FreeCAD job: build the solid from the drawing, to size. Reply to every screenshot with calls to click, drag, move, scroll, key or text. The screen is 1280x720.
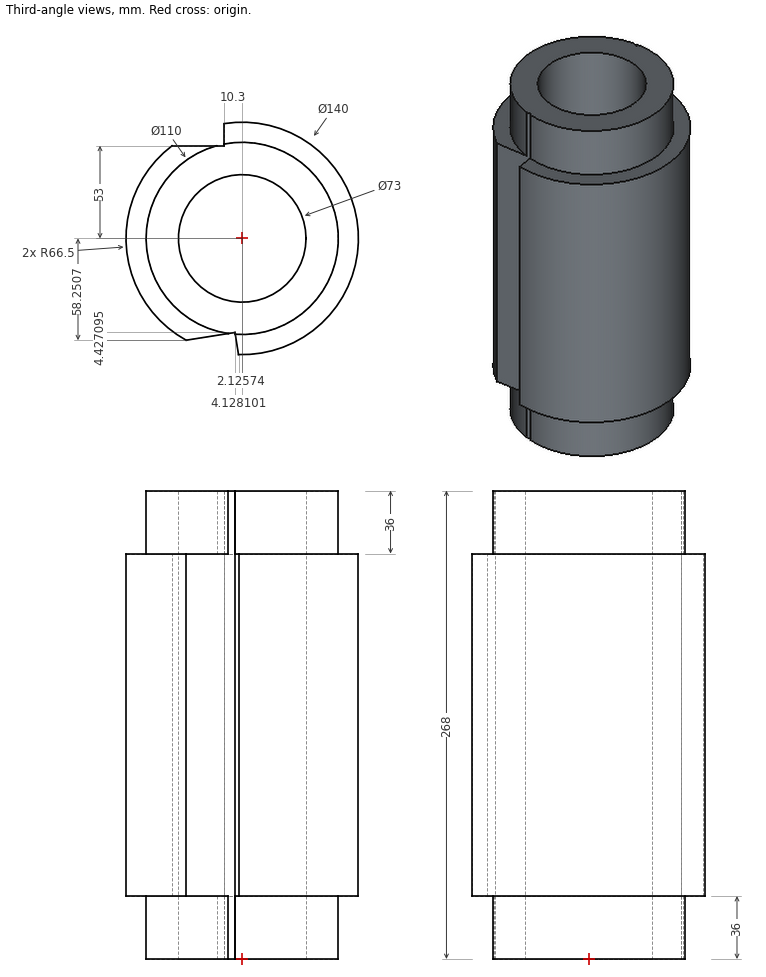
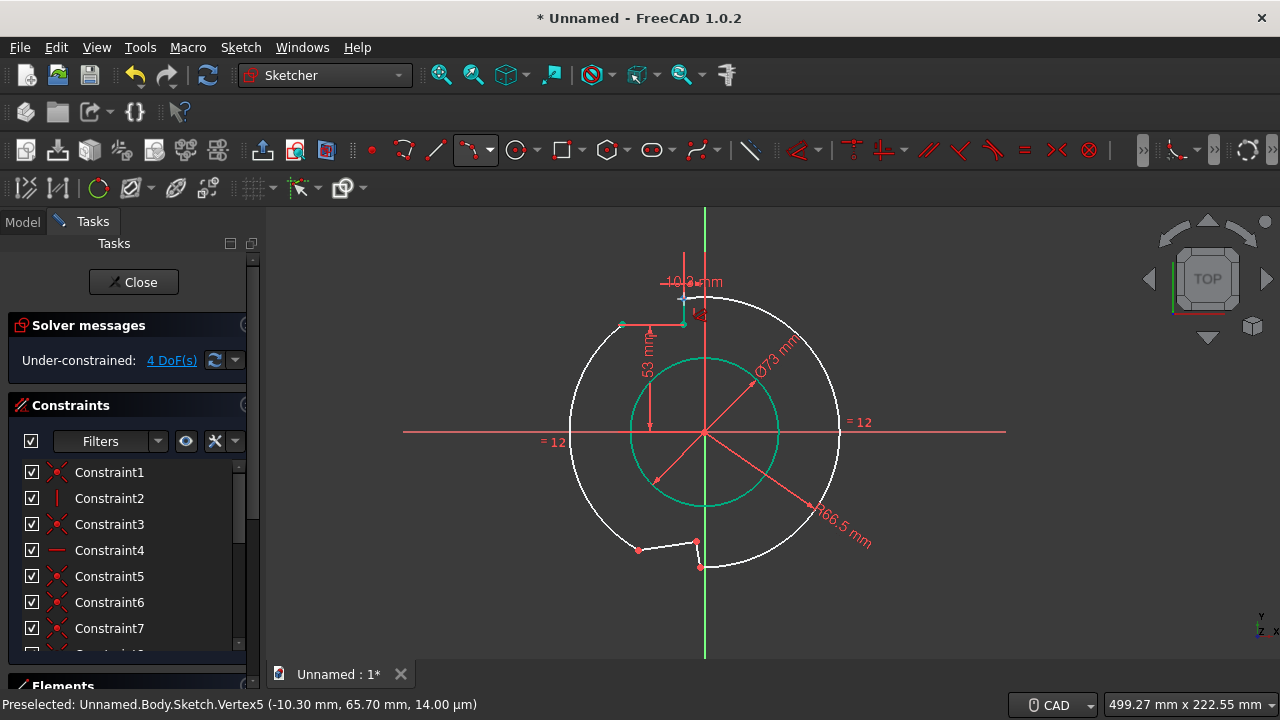
click(639, 550)
click(605, 491)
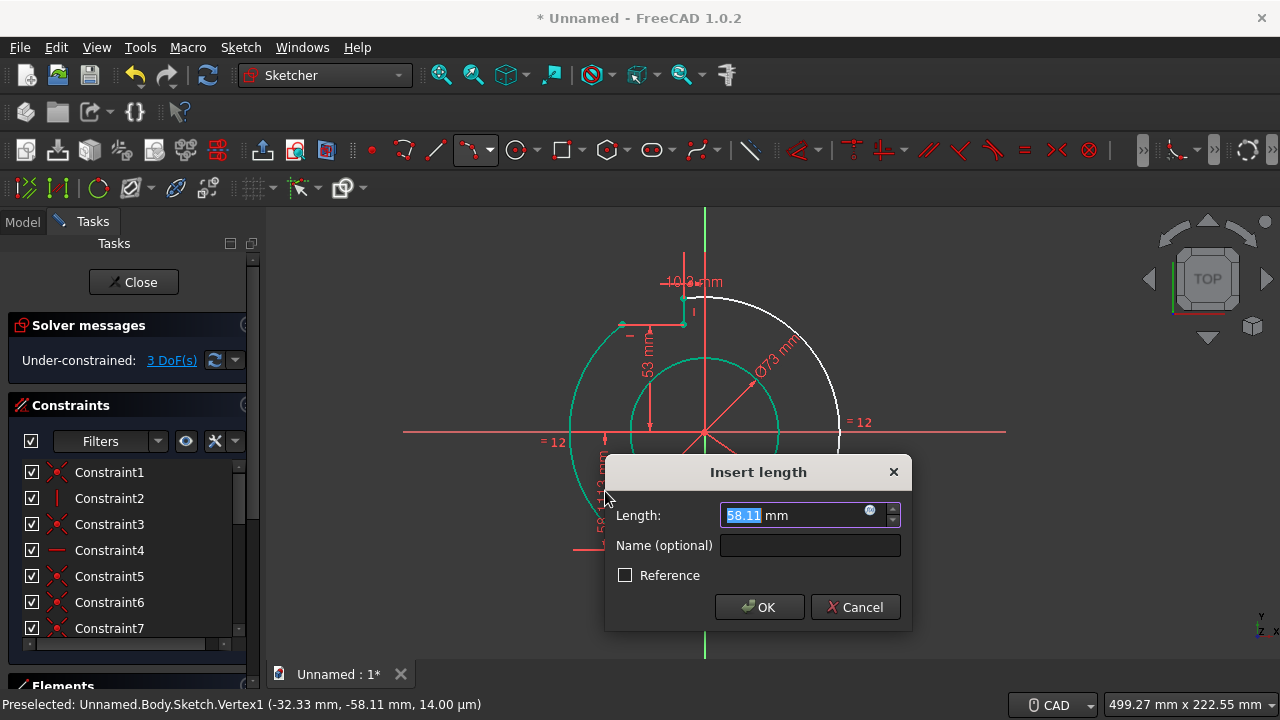
text(58.2507)
key(Return)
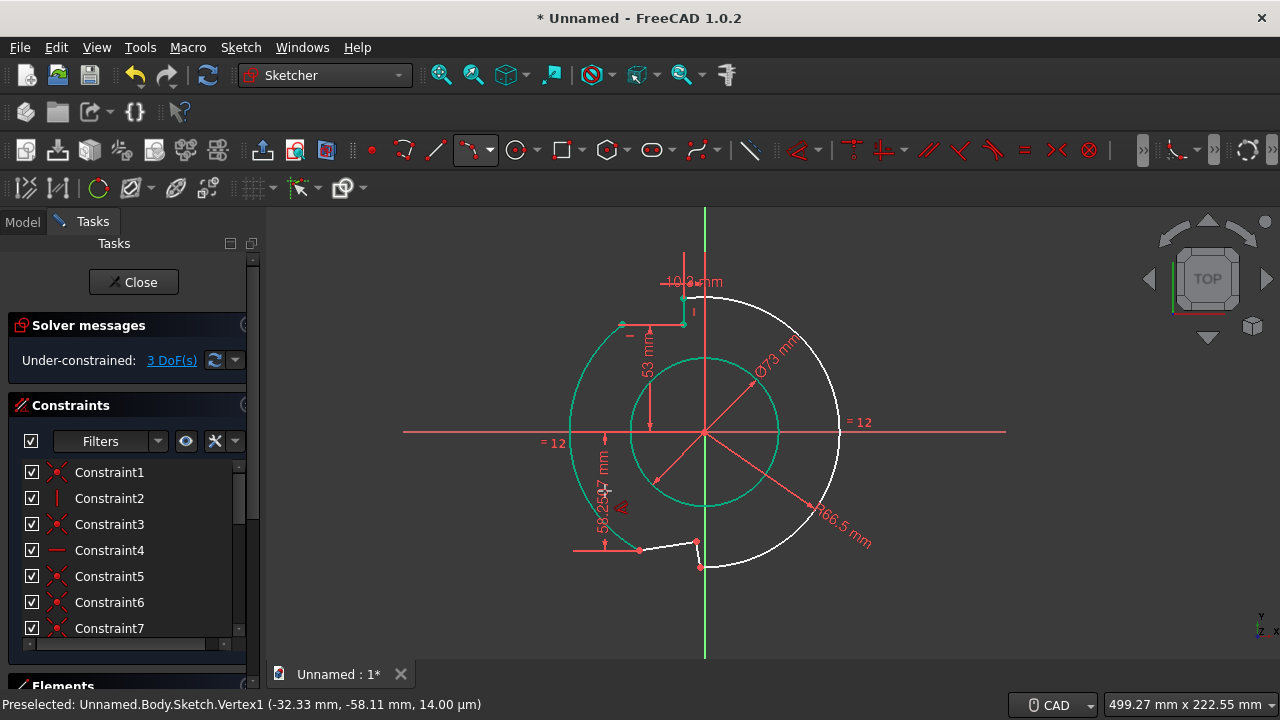
scroll(700, 567, up, 12)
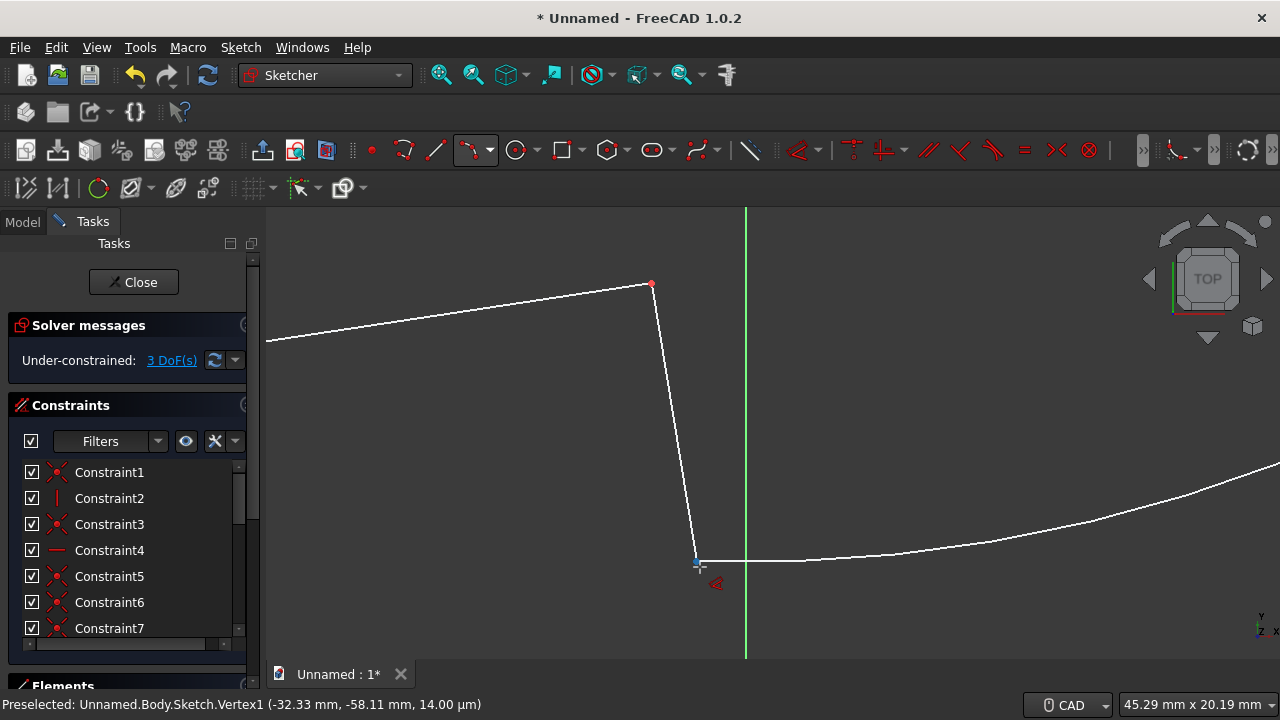
click(697, 561)
click(721, 595)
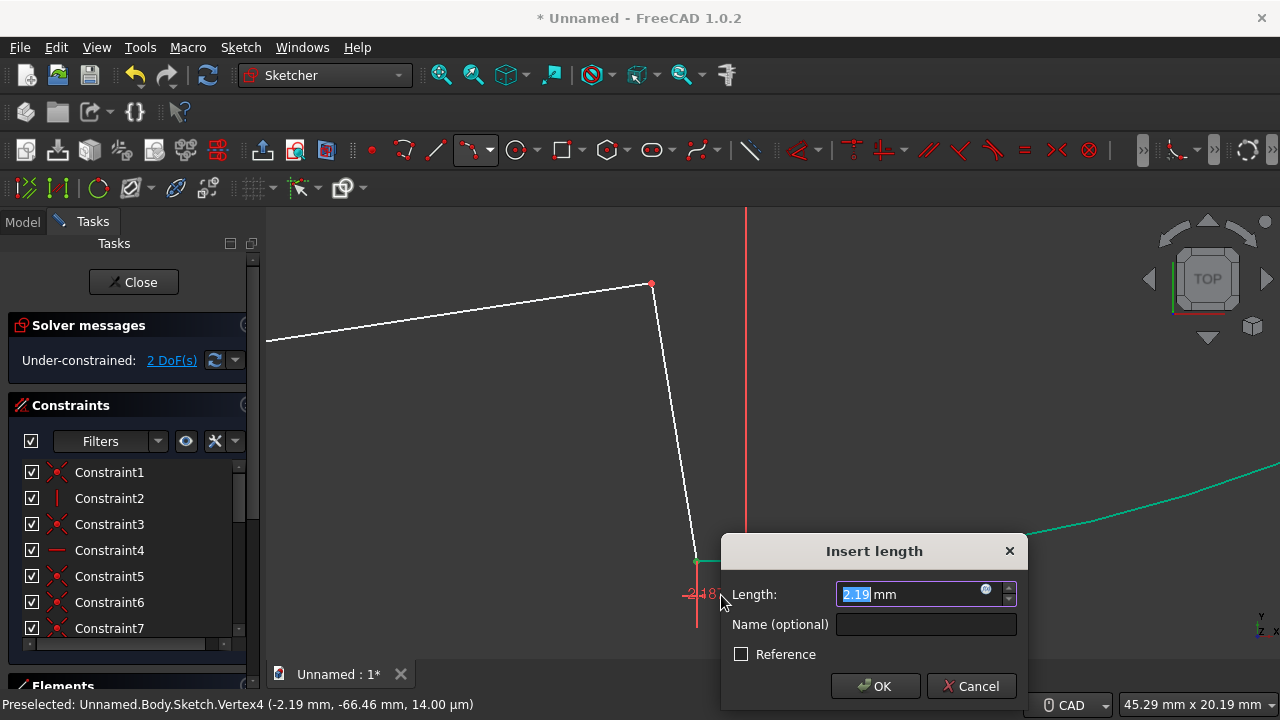
text(2.12574)
key(Return)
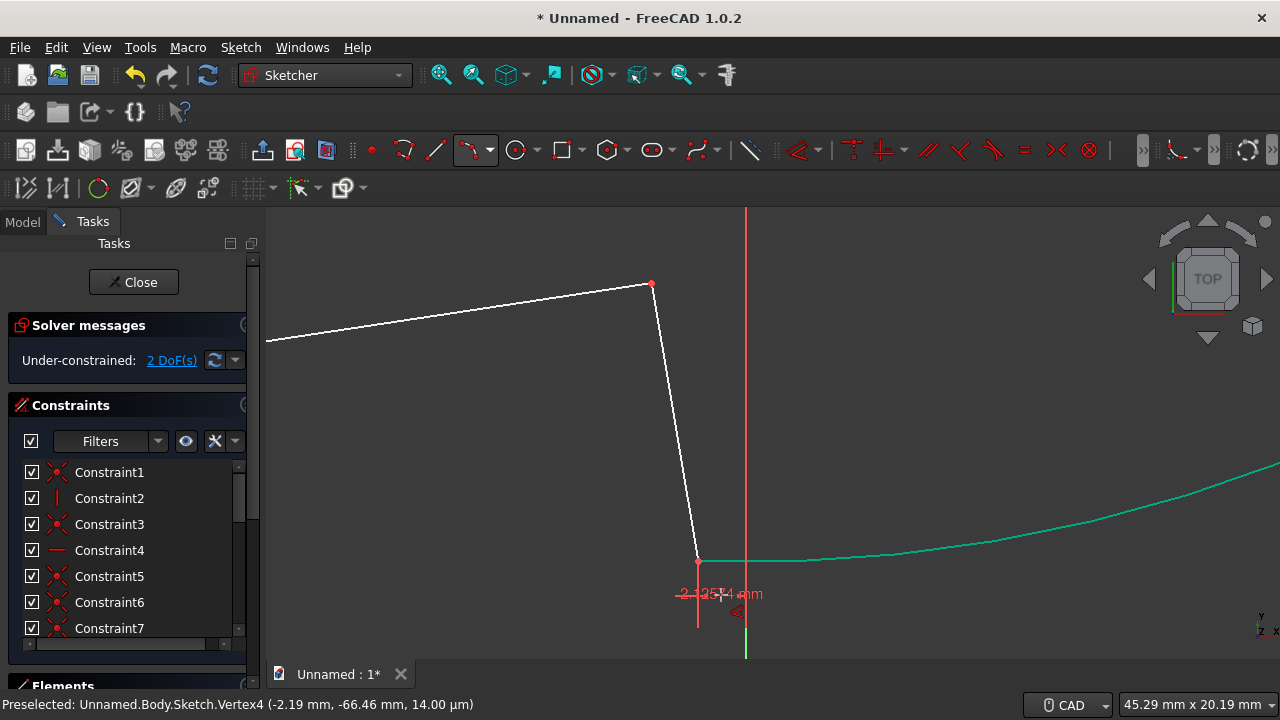
click(652, 283)
click(699, 317)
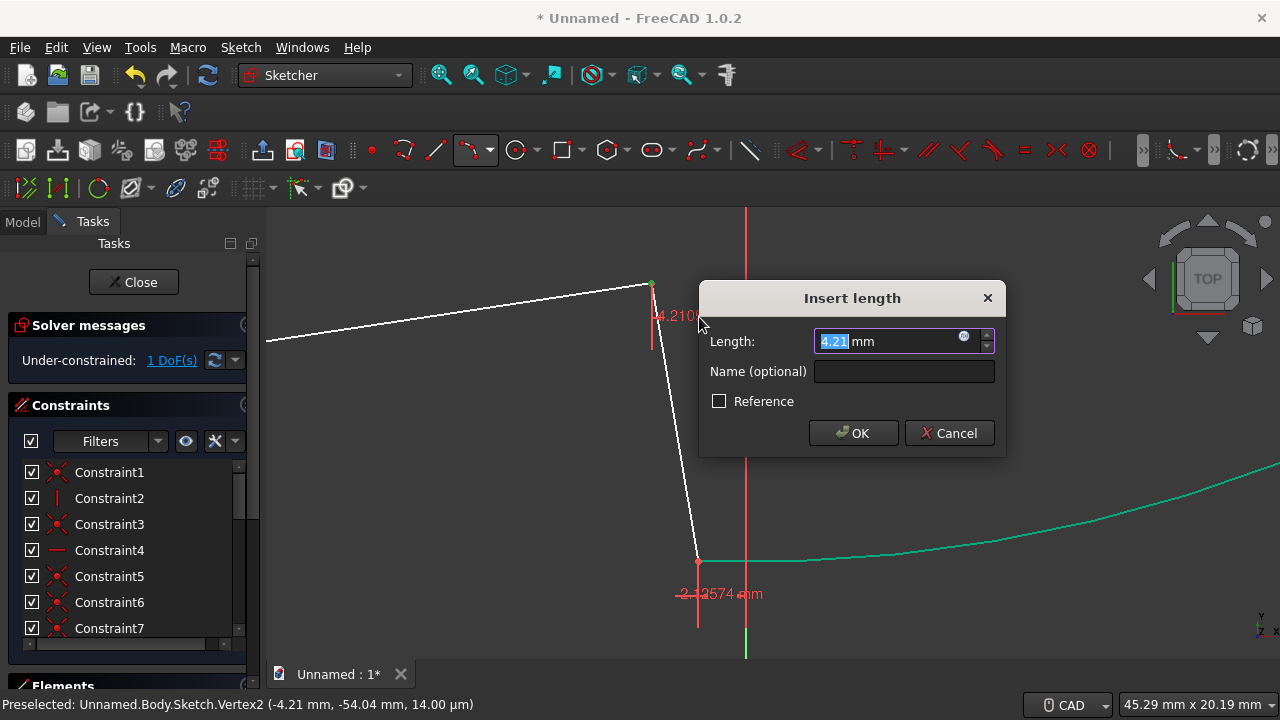
text(4.128101)
key(Return)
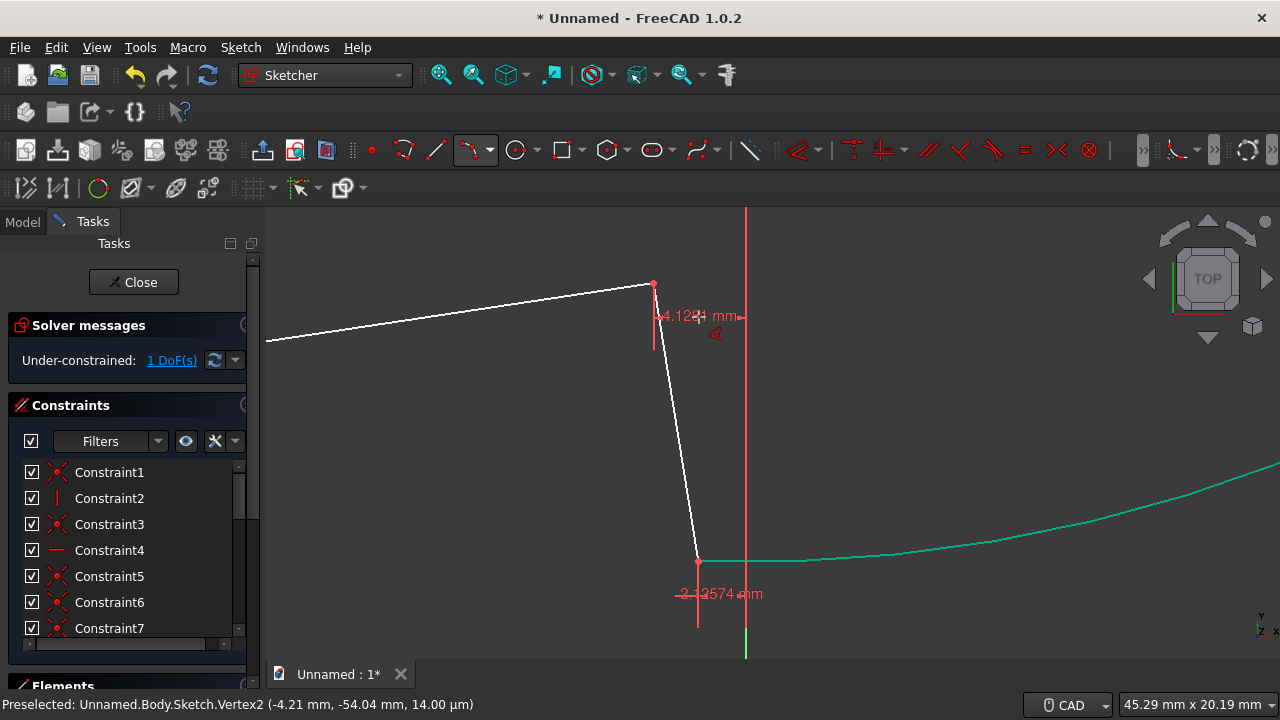
click(466, 311)
click(688, 352)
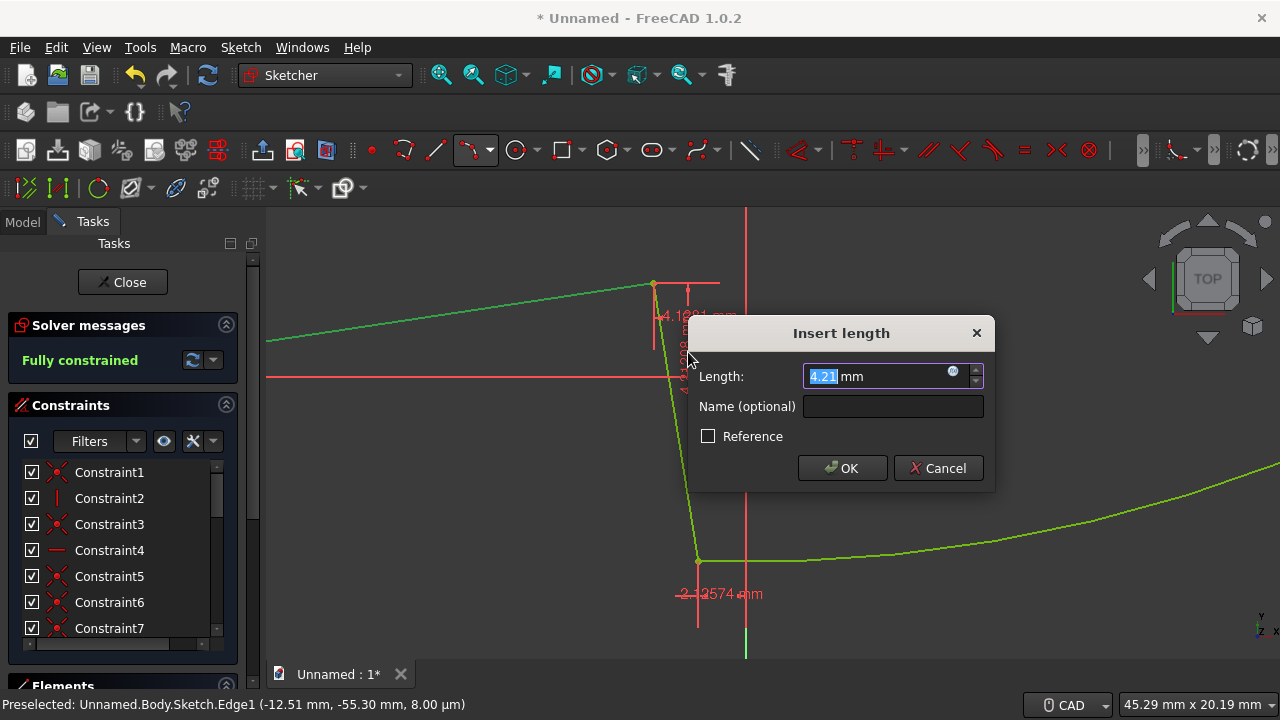
text(4.427095)
key(Return)
key(Escape)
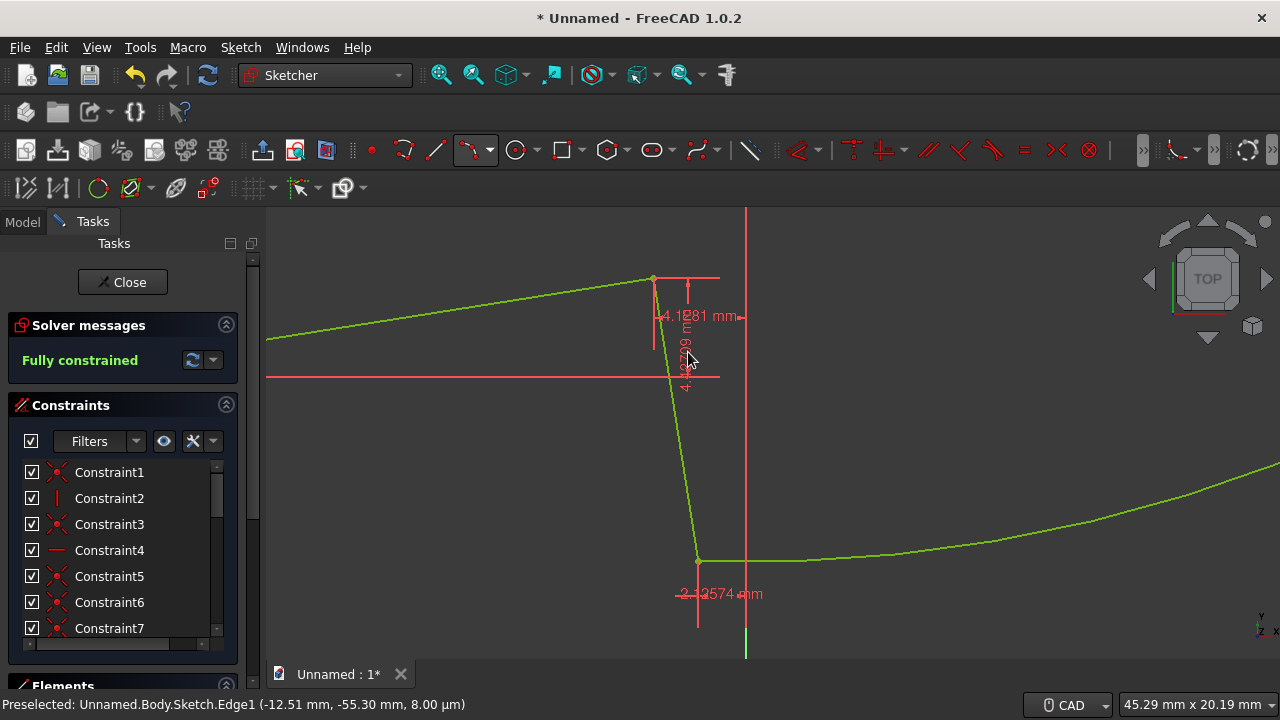
click(123, 282)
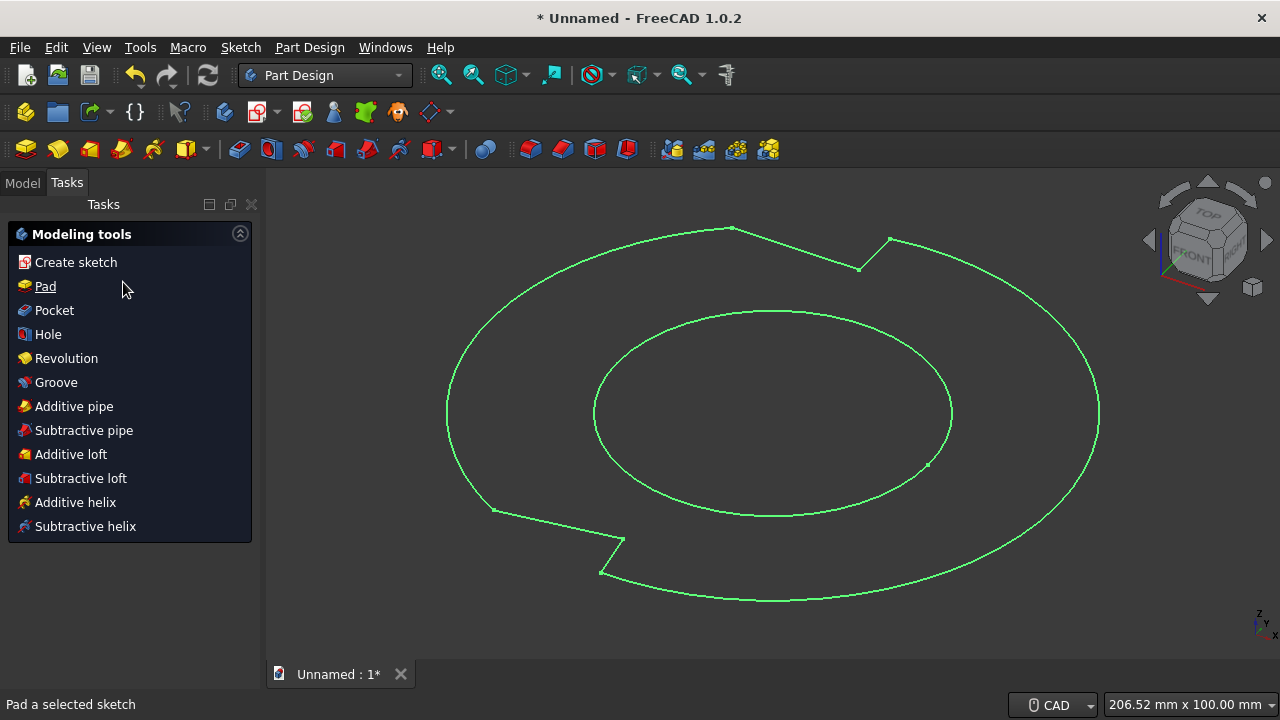
click(26, 150)